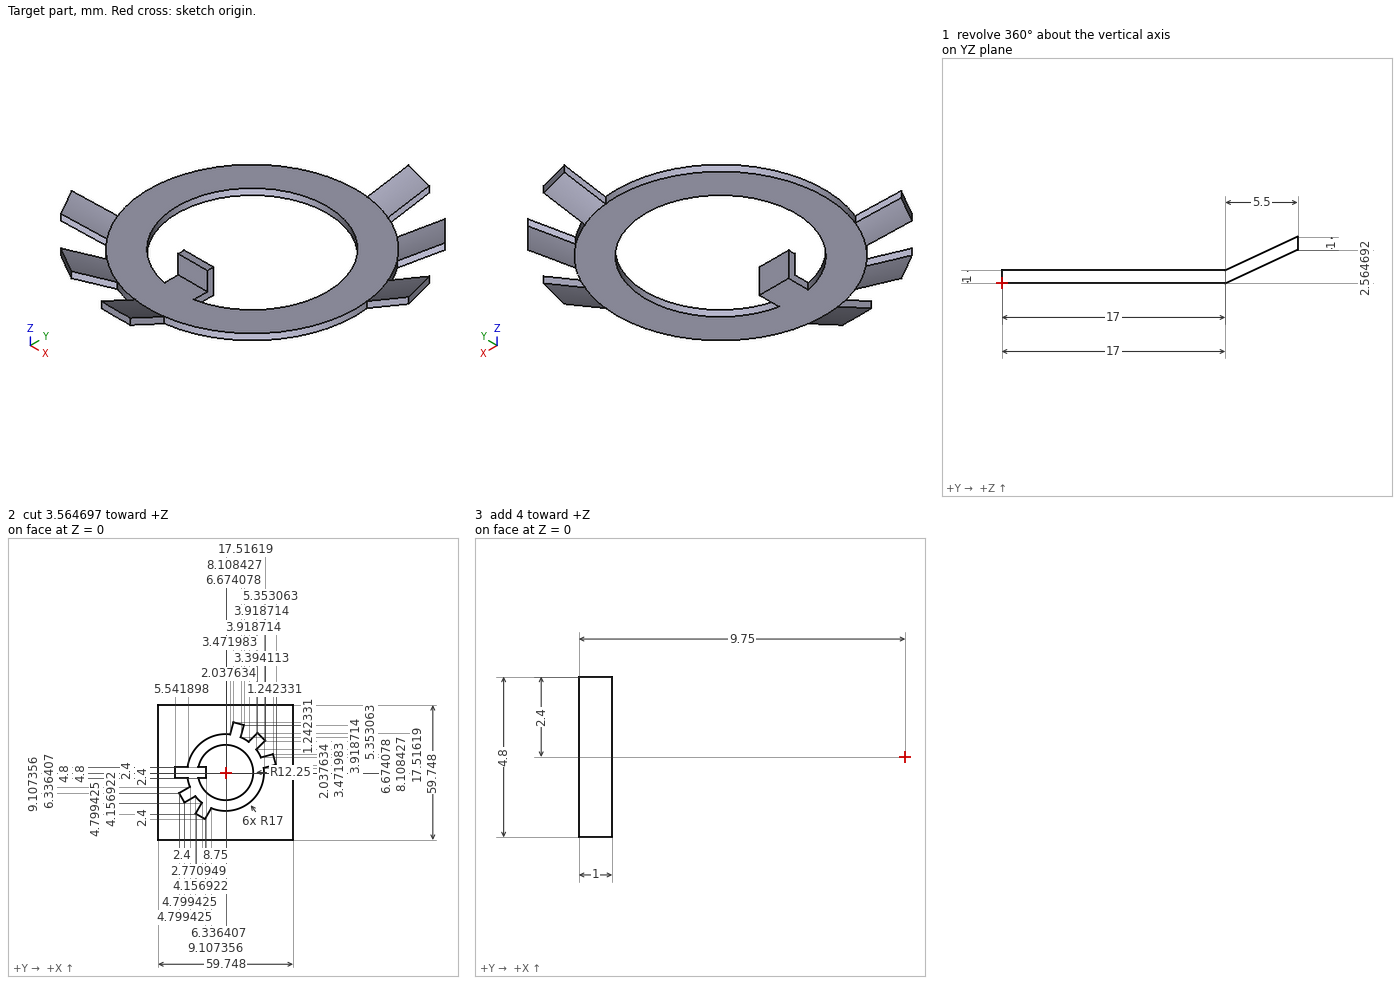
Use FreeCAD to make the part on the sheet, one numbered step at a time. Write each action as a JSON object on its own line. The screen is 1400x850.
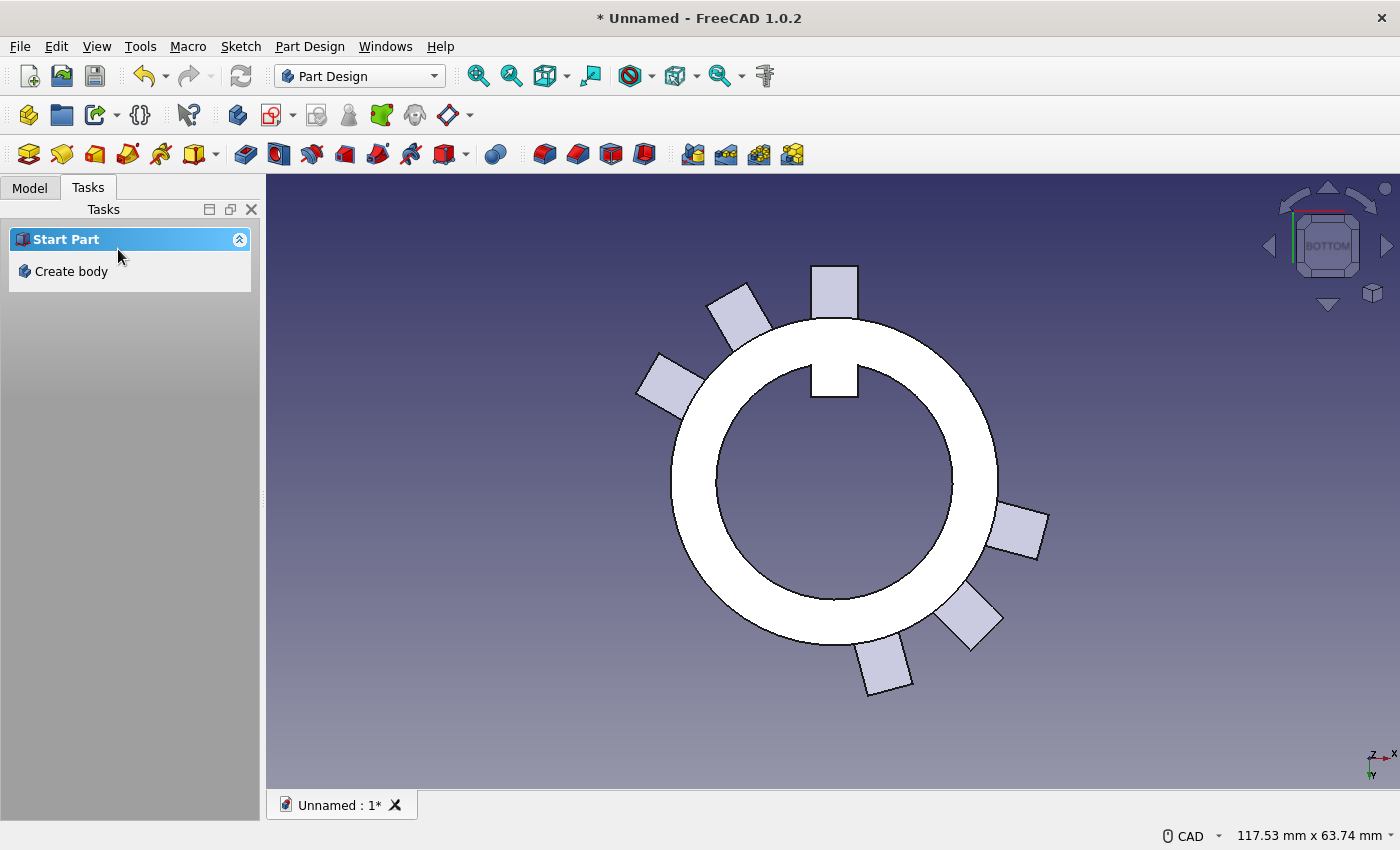
{"action": "key", "text": "0"}